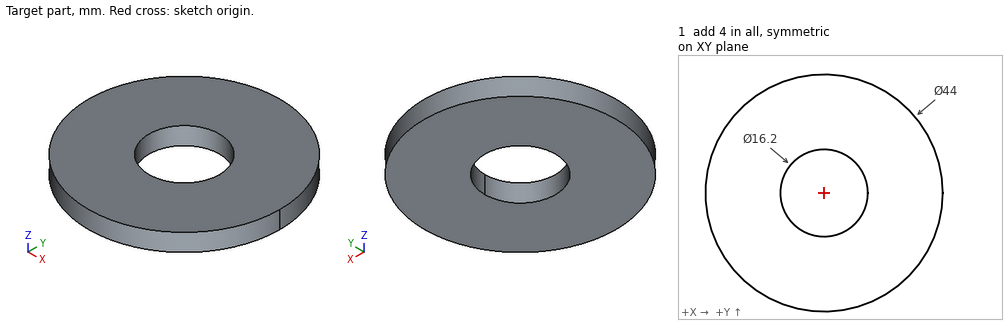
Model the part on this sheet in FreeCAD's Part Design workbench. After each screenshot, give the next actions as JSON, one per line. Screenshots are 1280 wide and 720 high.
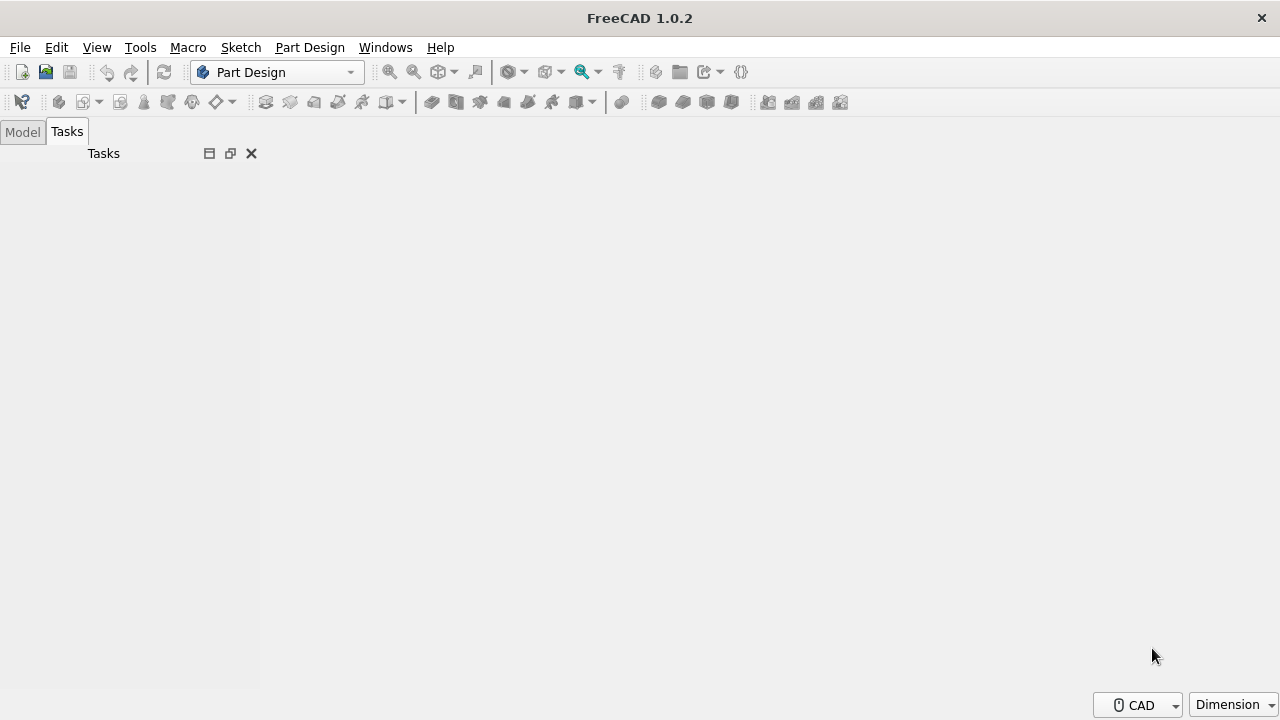
{"action": "key", "text": "ctrl+n"}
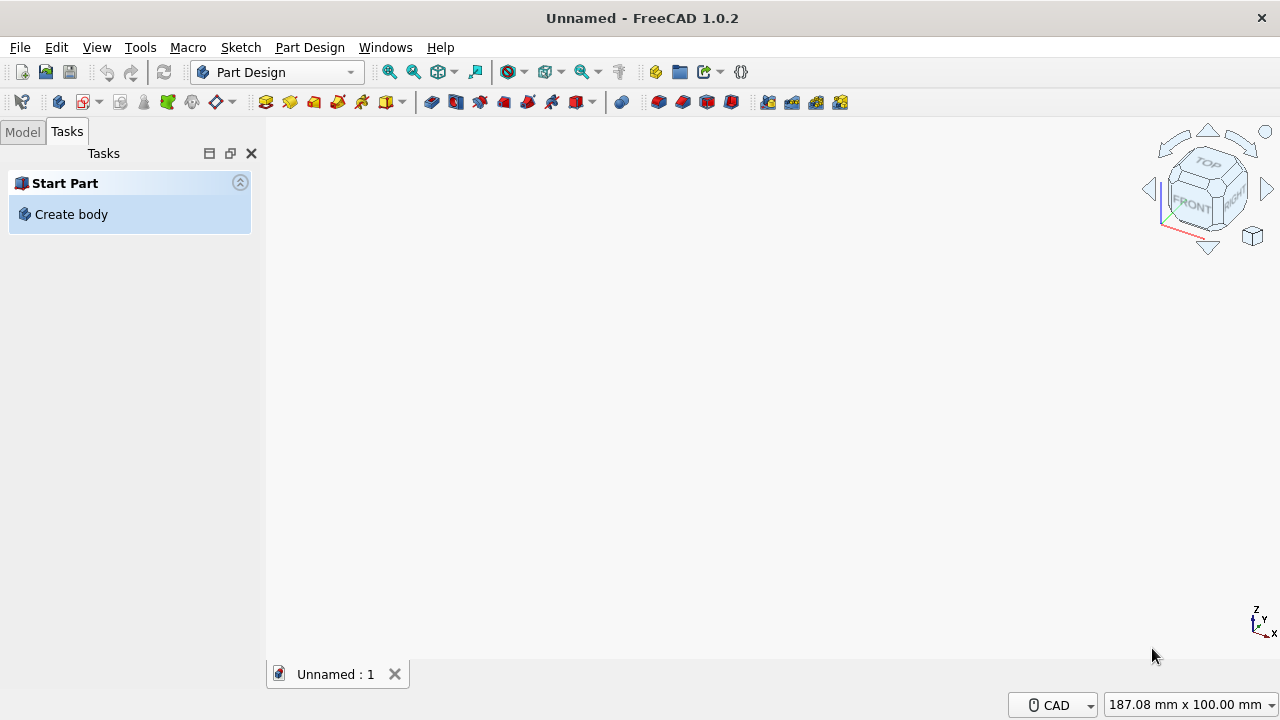
{"action": "left_click", "coordinate": [84, 102]}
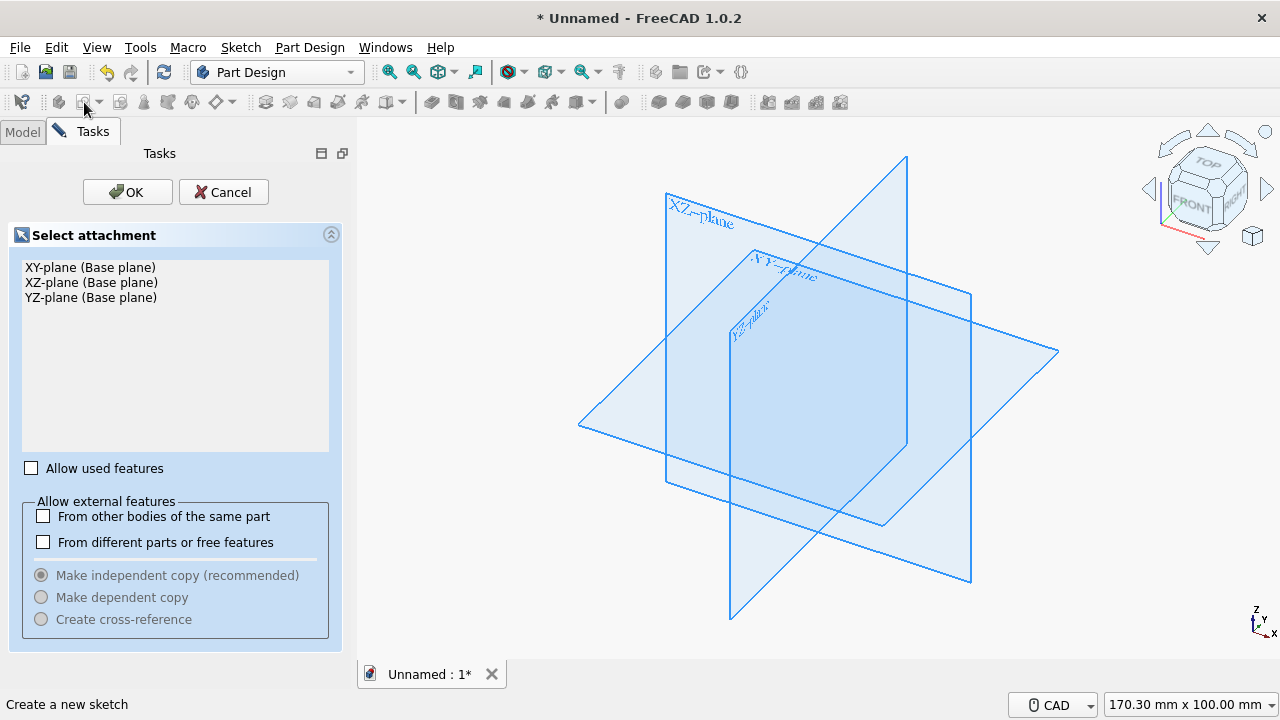
{"action": "left_click", "coordinate": [82, 268]}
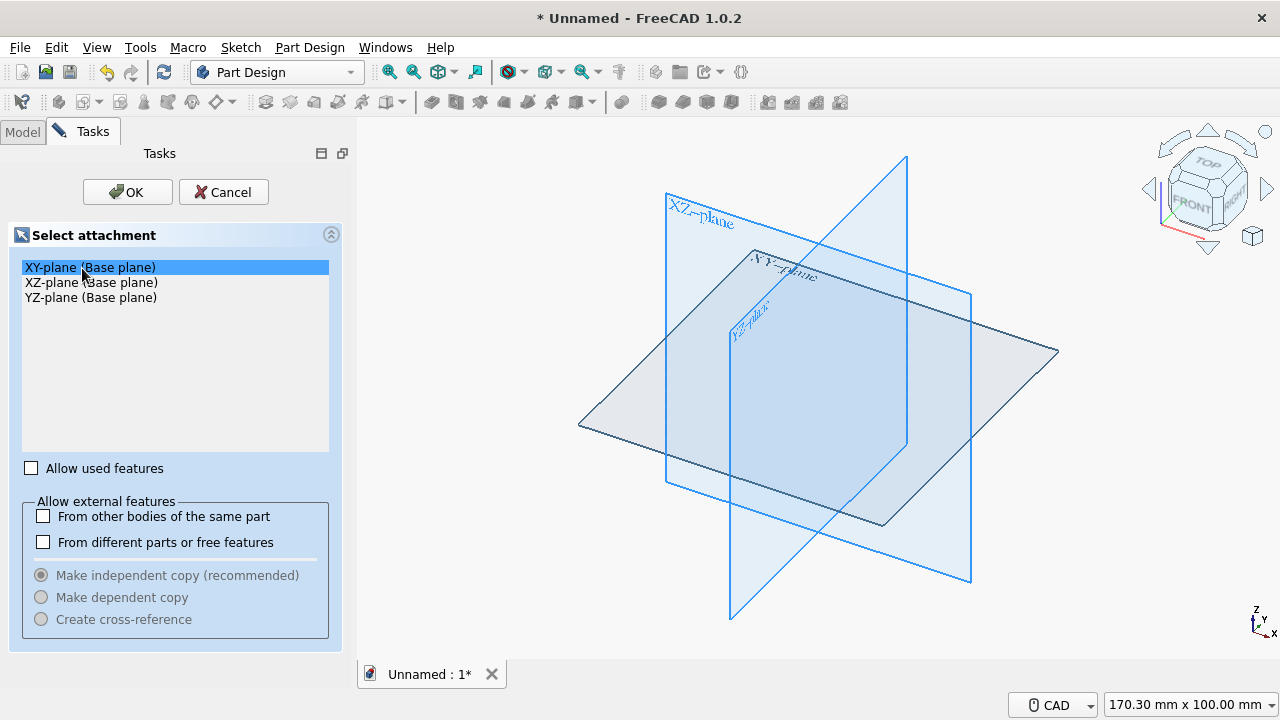
{"action": "left_click", "coordinate": [128, 192]}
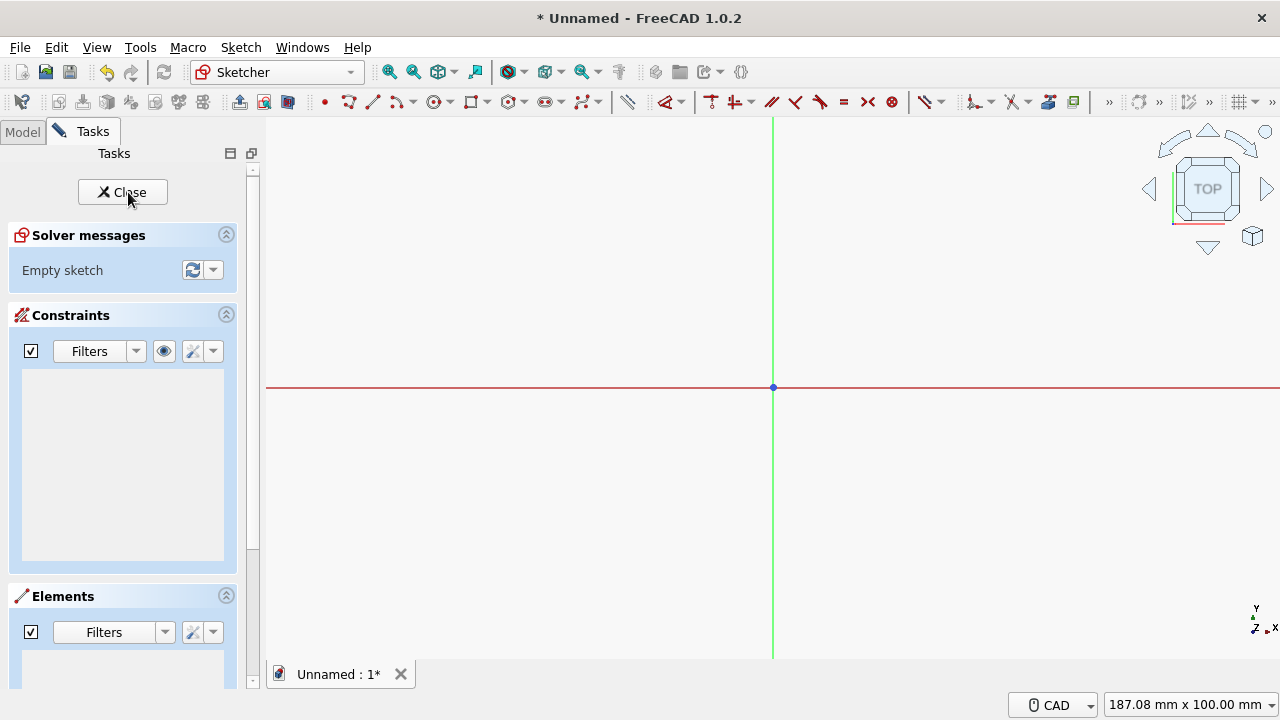
{"action": "scroll", "coordinate": [912, 388], "scroll_direction": "up", "scroll_amount": 2}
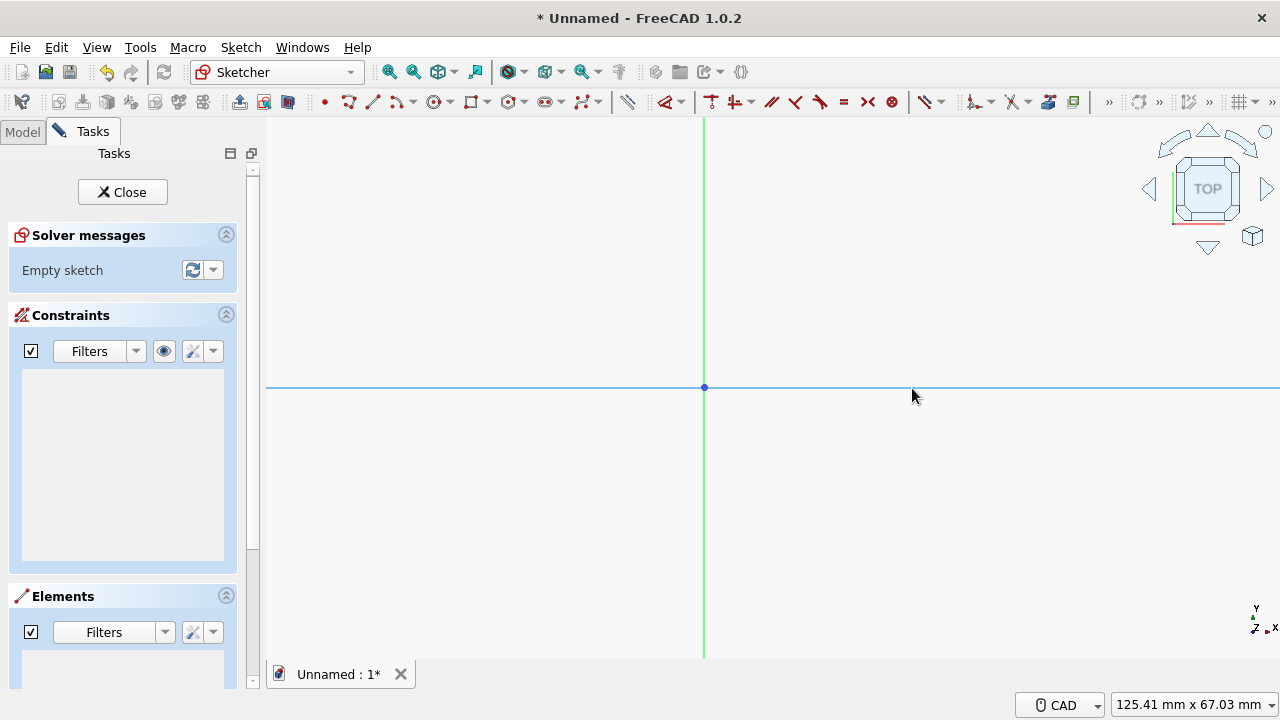
{"action": "key", "text": "g c"}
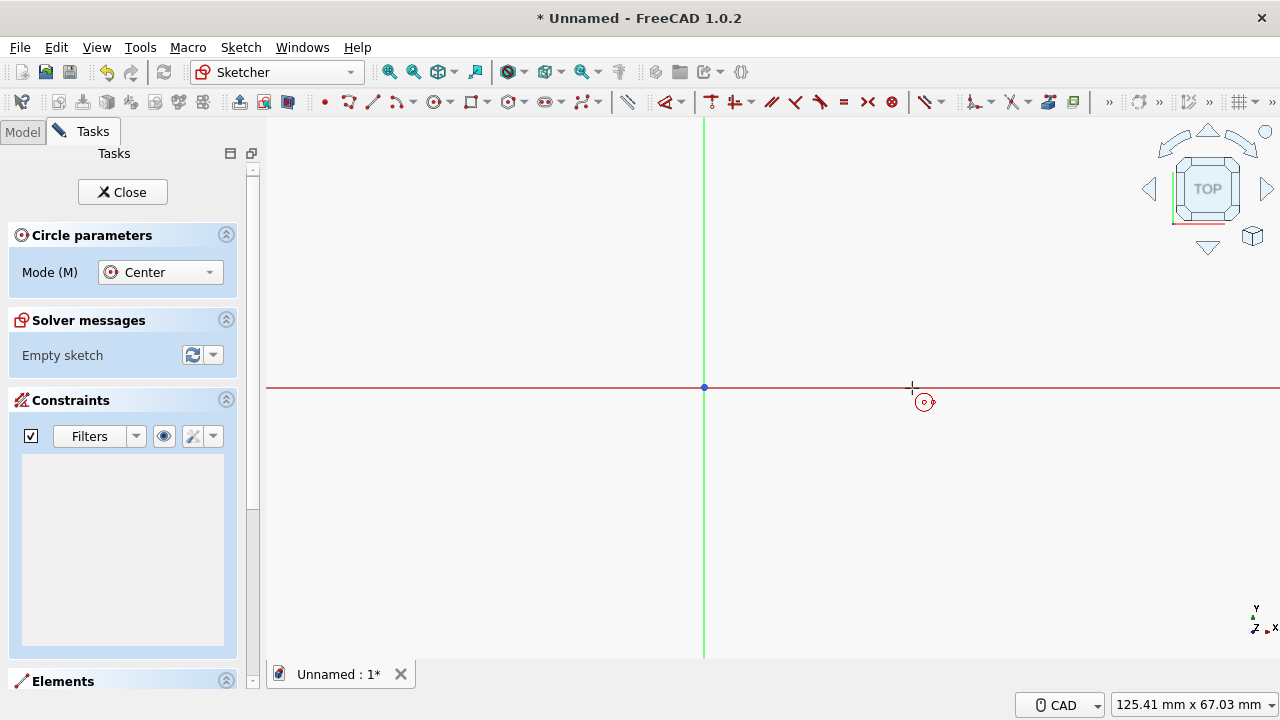
{"action": "left_click", "coordinate": [704, 388]}
{"action": "mouse_move", "coordinate": [830, 262]}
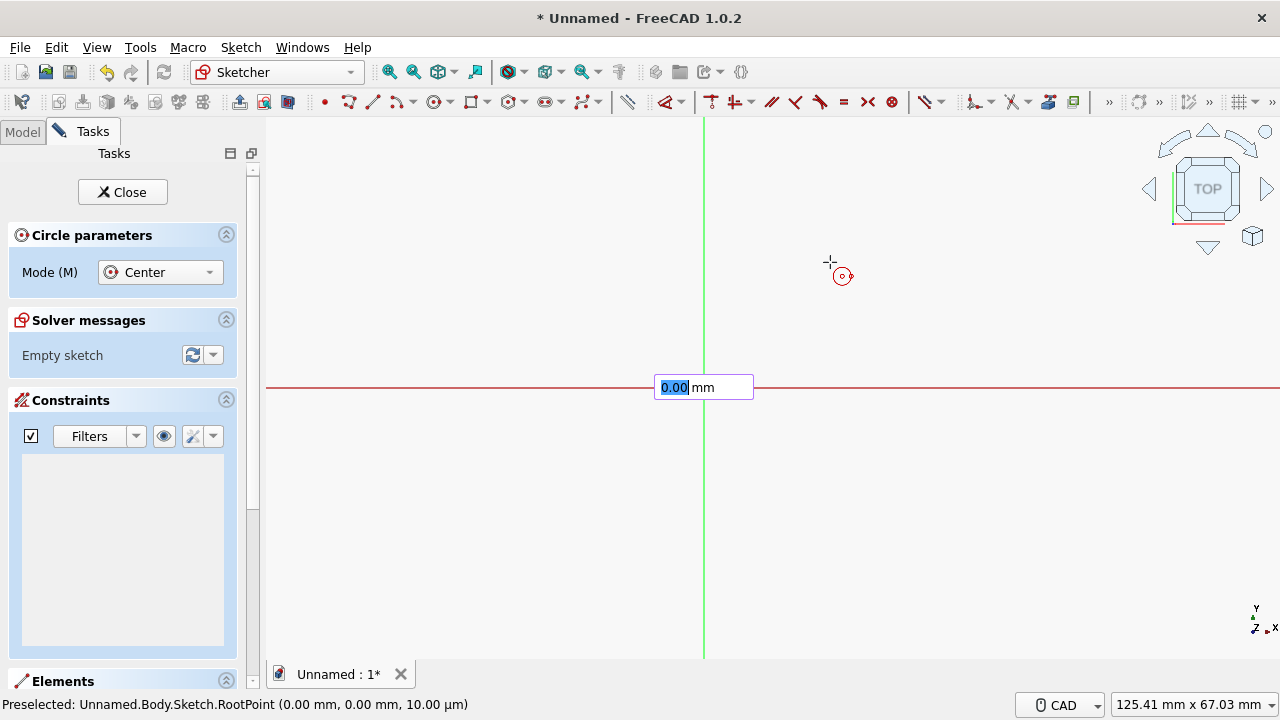
{"action": "type", "text": "44"}
{"action": "key", "text": "Return"}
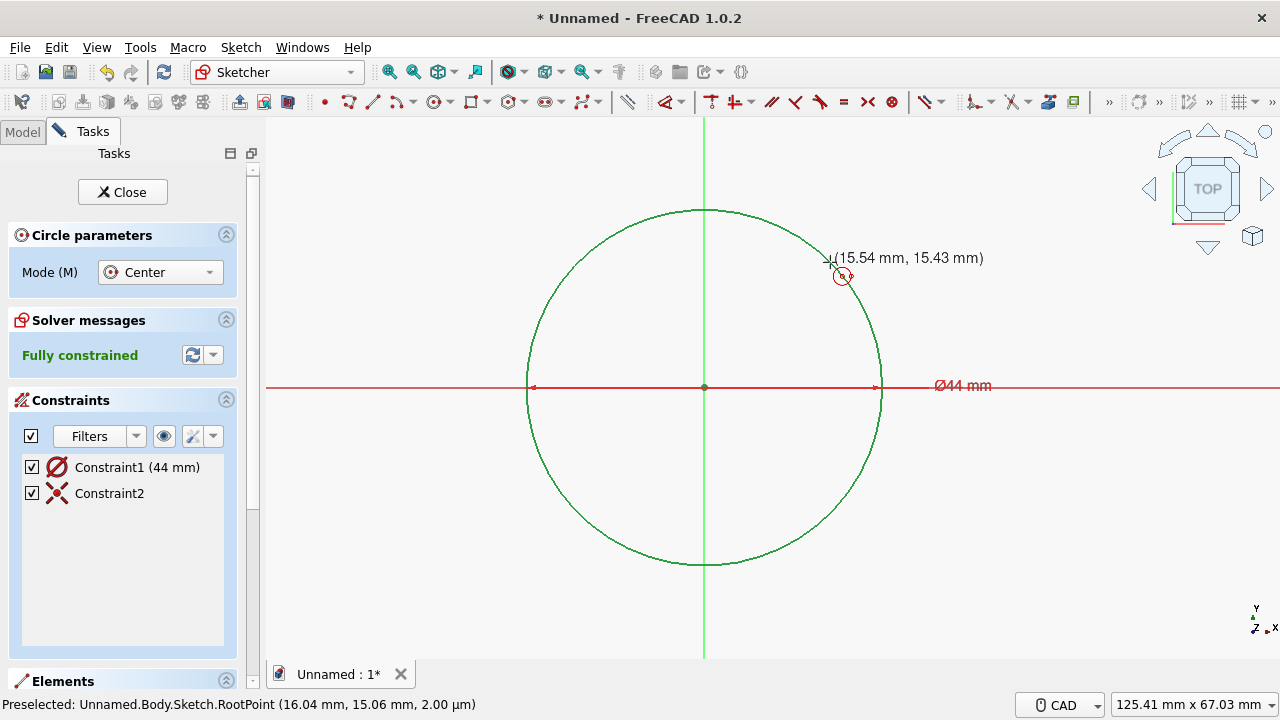
{"action": "left_click", "coordinate": [704, 388]}
{"action": "mouse_move", "coordinate": [751, 341]}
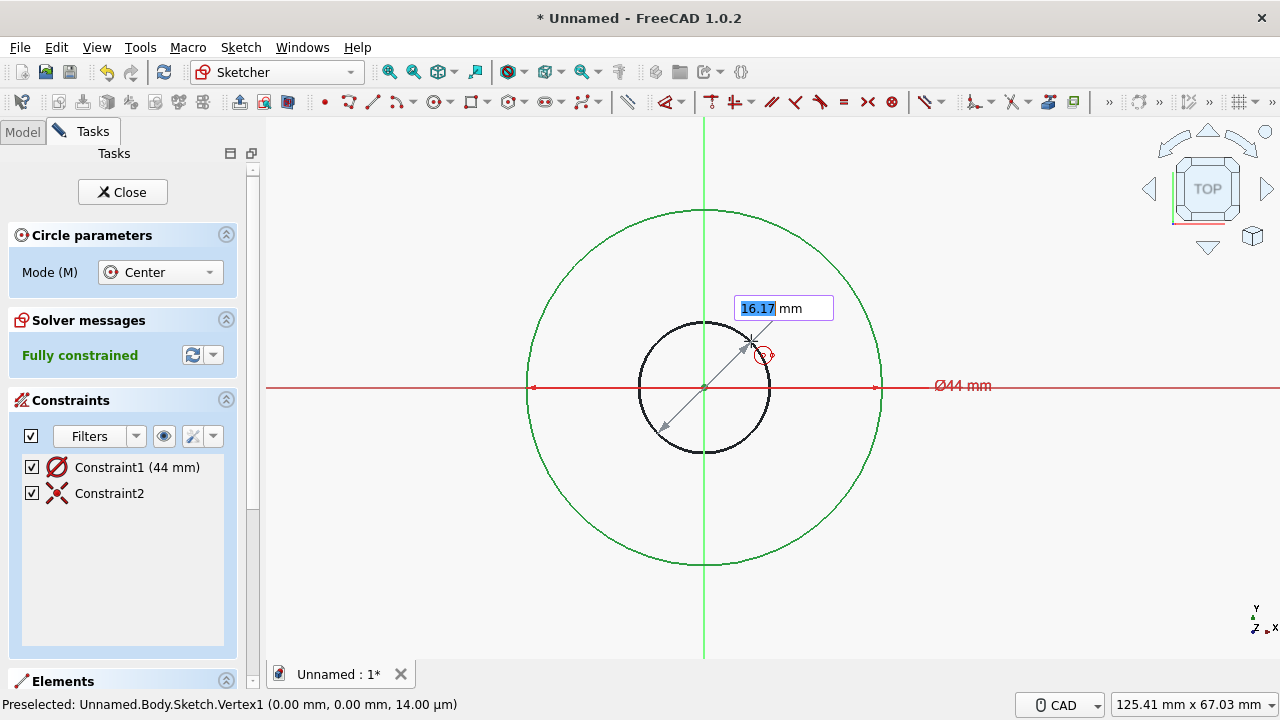
{"action": "type", "text": "16.2"}
{"action": "key", "text": "Return"}
{"action": "key", "text": "Escape"}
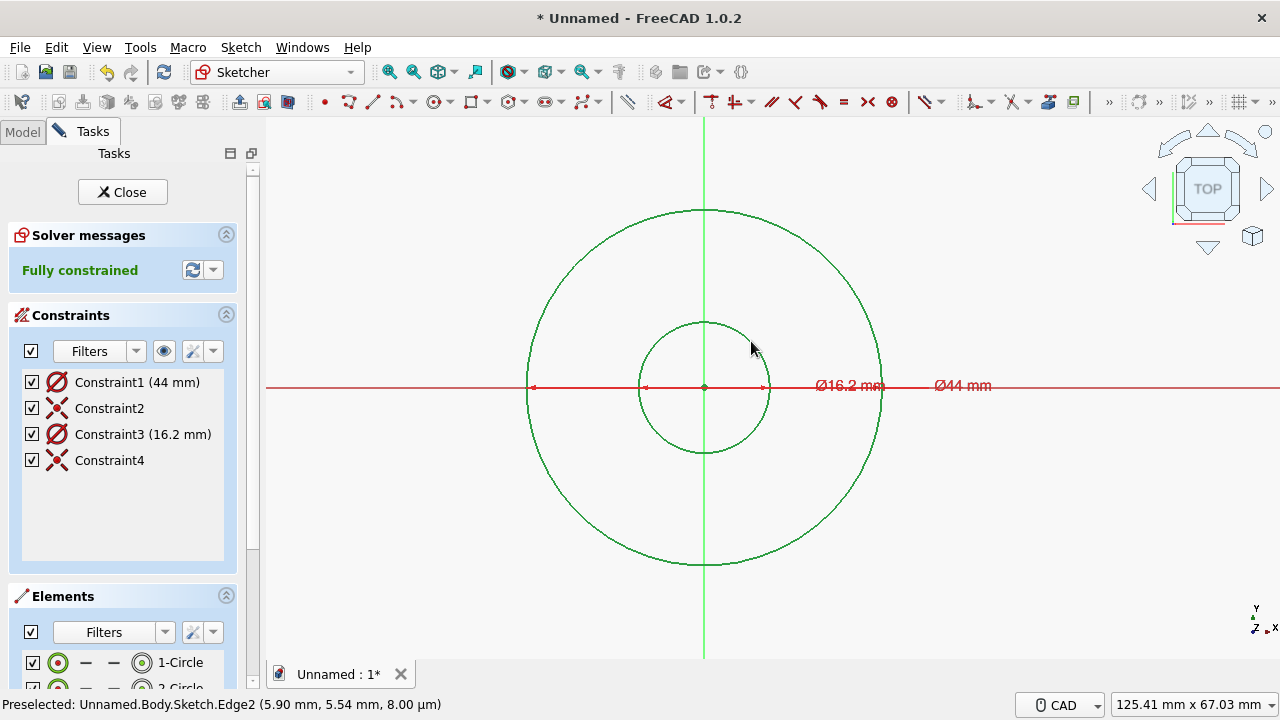
{"action": "left_click", "coordinate": [123, 192]}